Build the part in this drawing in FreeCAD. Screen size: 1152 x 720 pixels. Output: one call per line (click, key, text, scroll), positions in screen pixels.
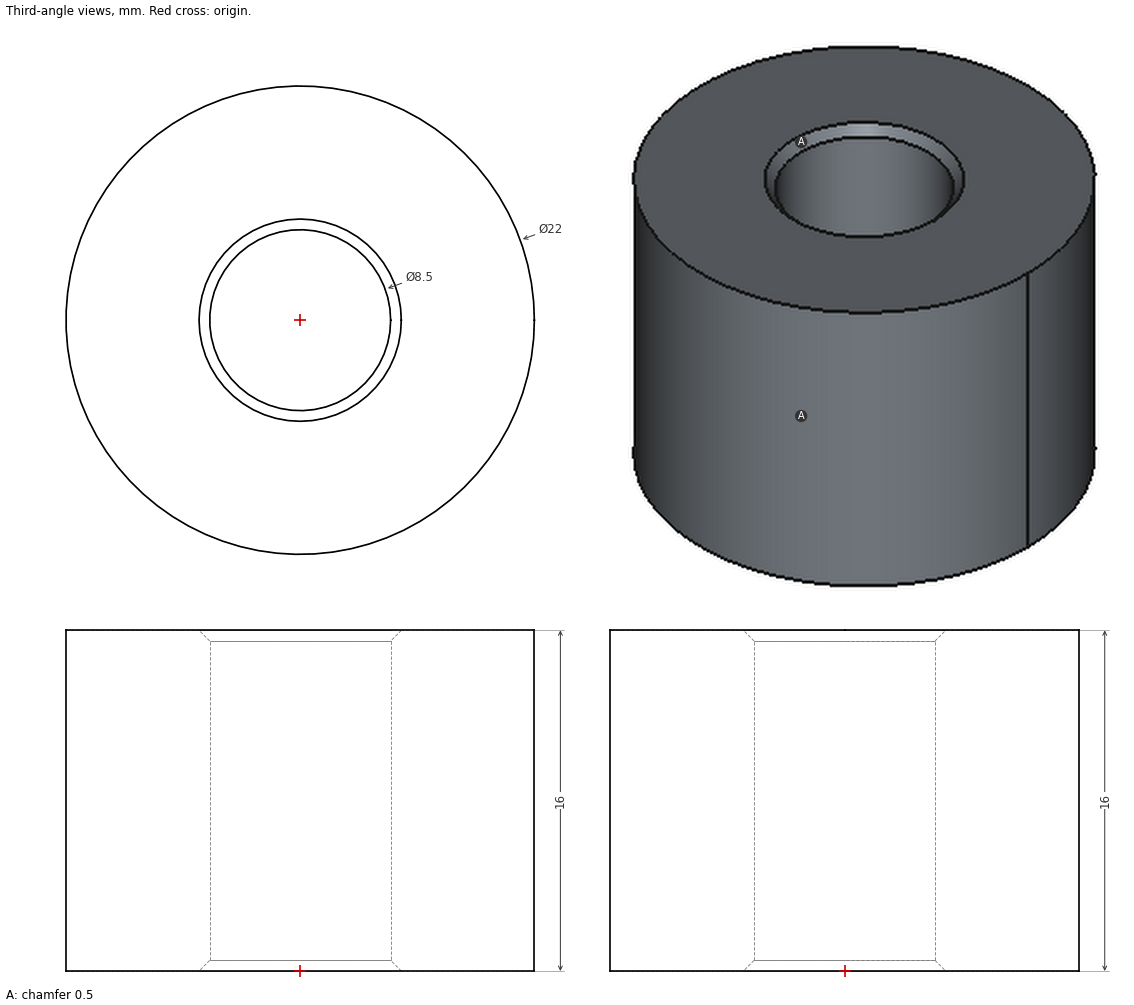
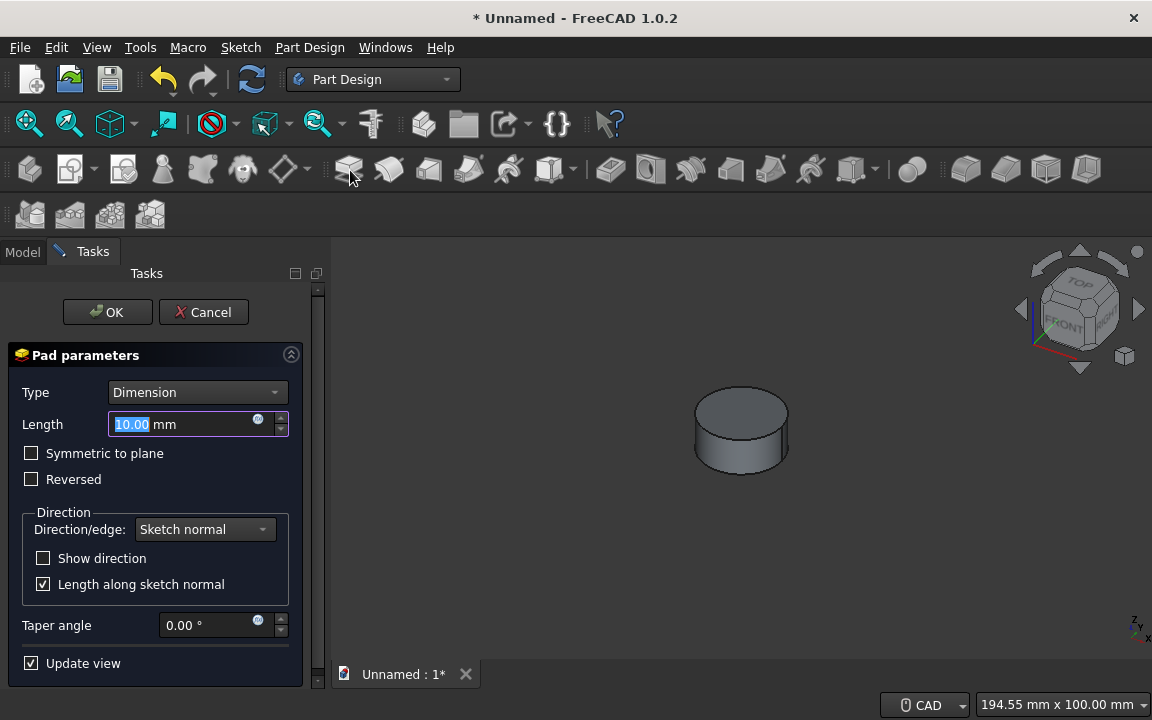
text(16)
key(Tab)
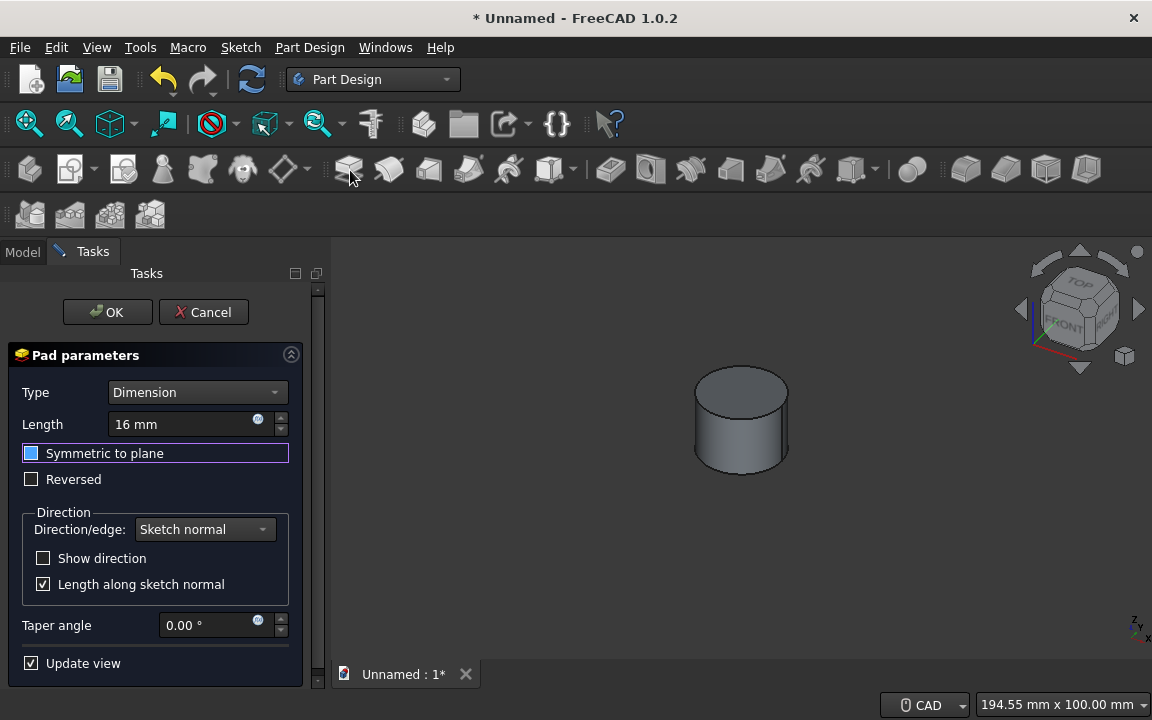
click(108, 312)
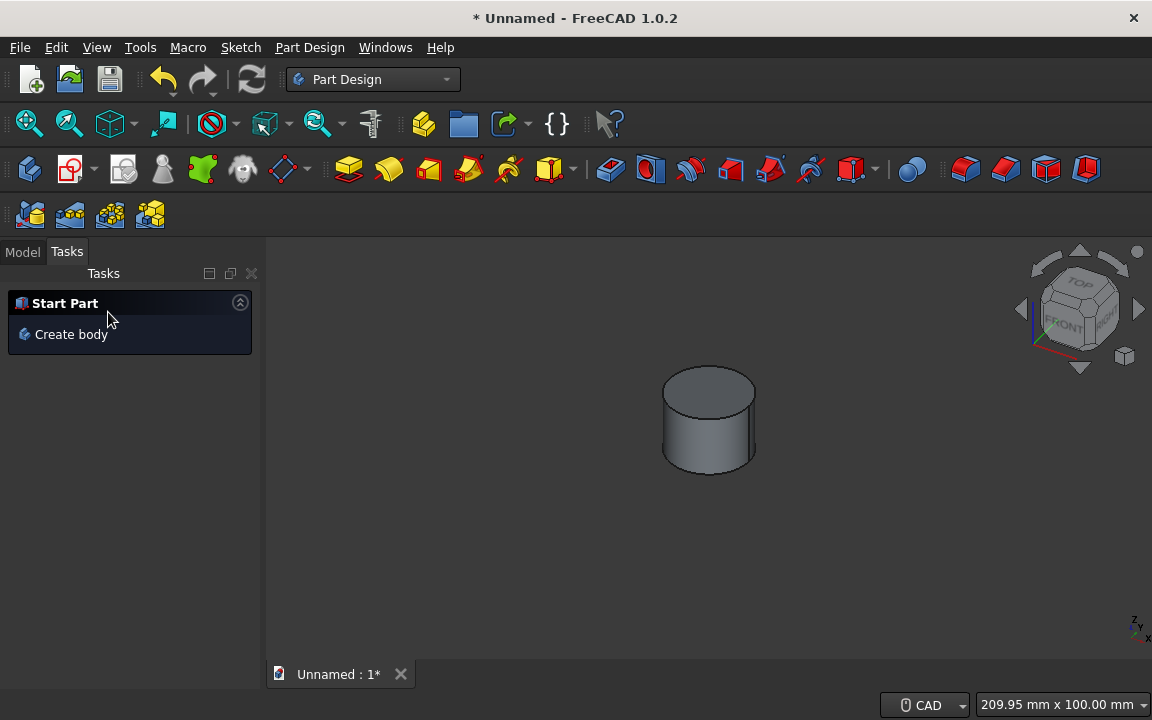
key(v)
key(f)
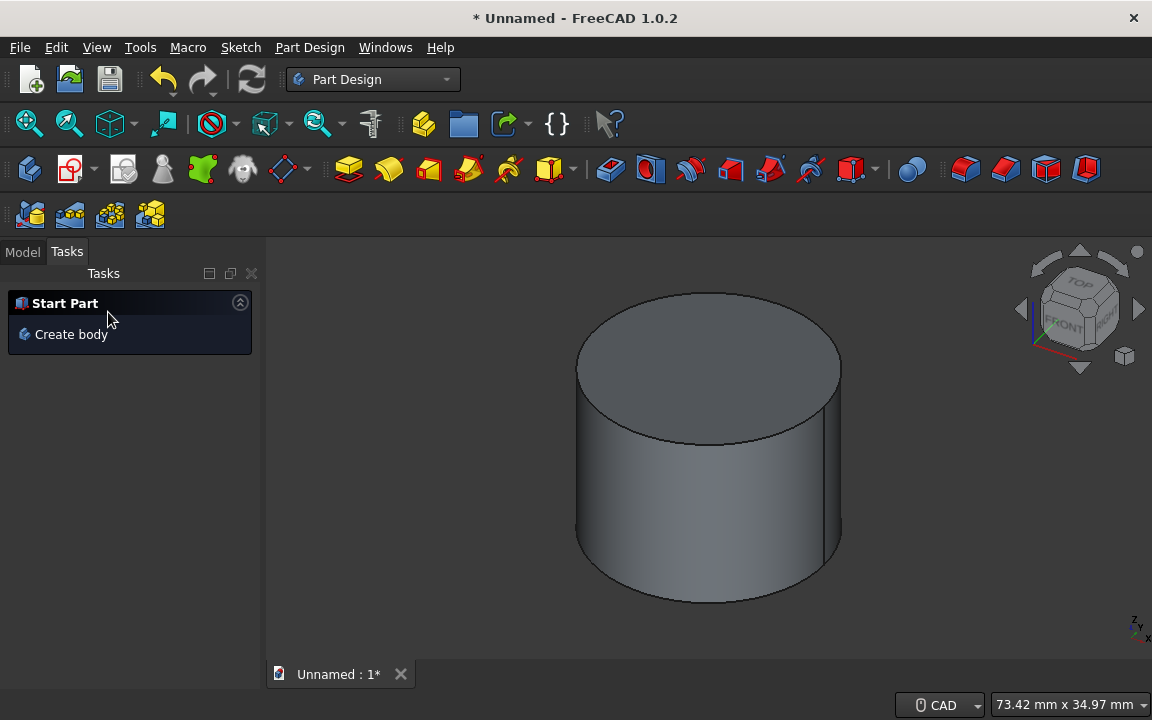
click(709, 368)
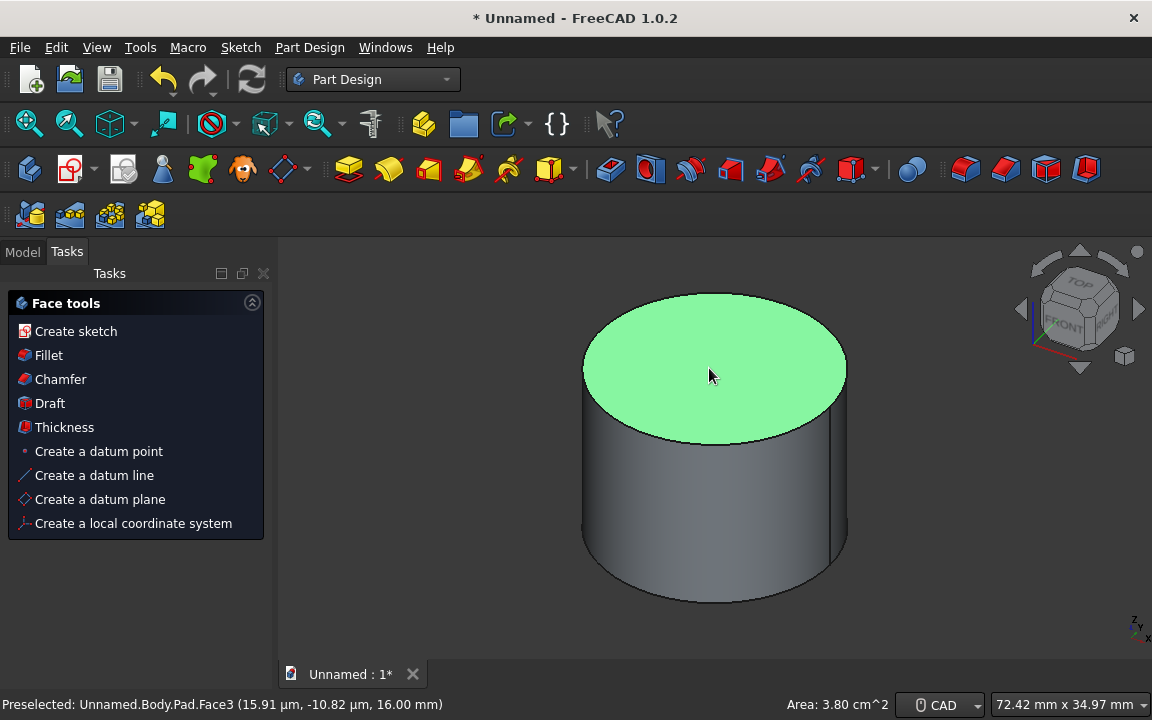
click(70, 170)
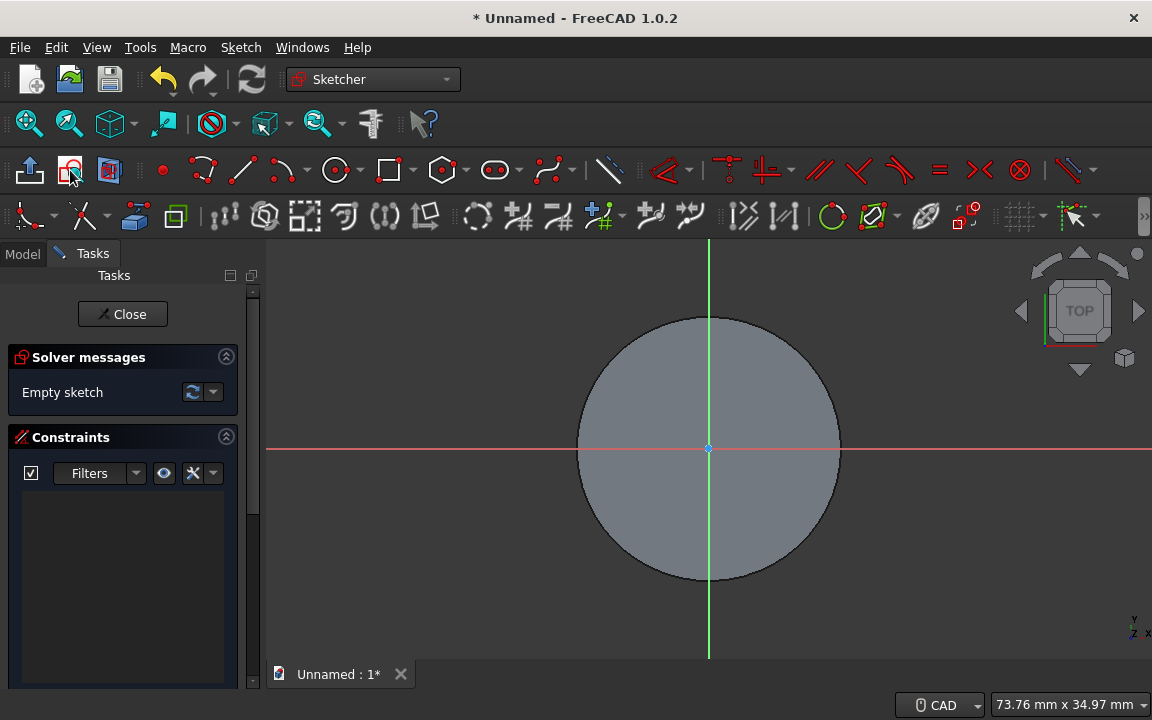
scroll(749, 449, up, 5)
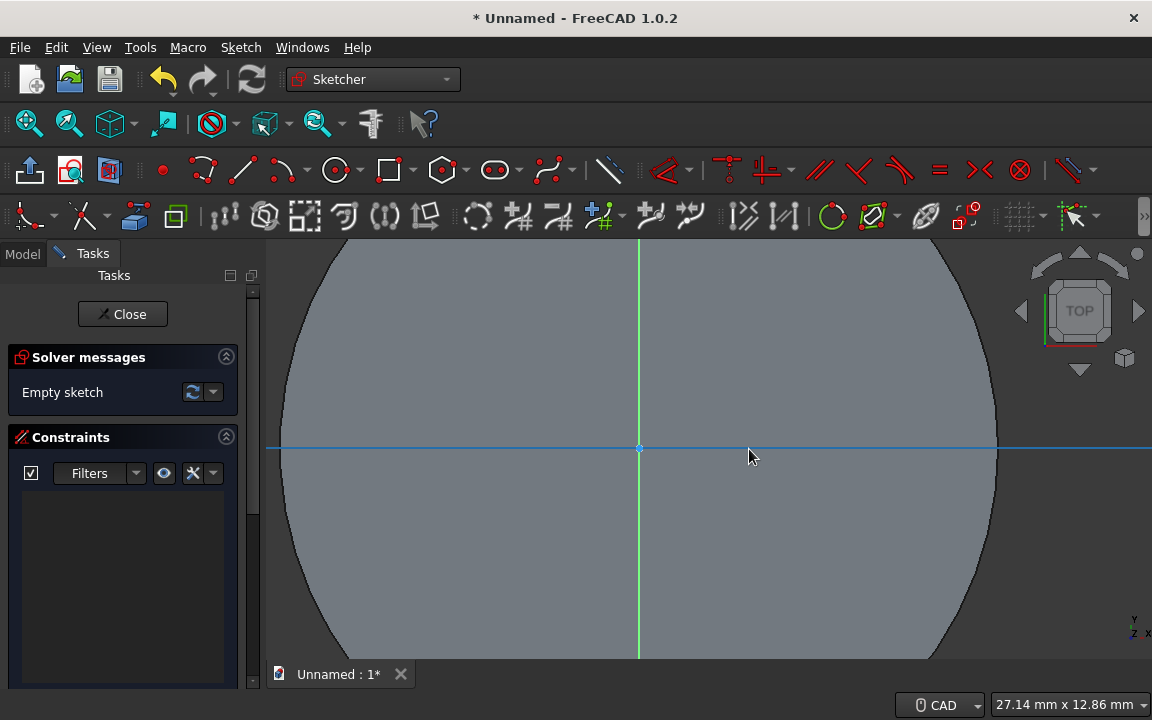
click(336, 170)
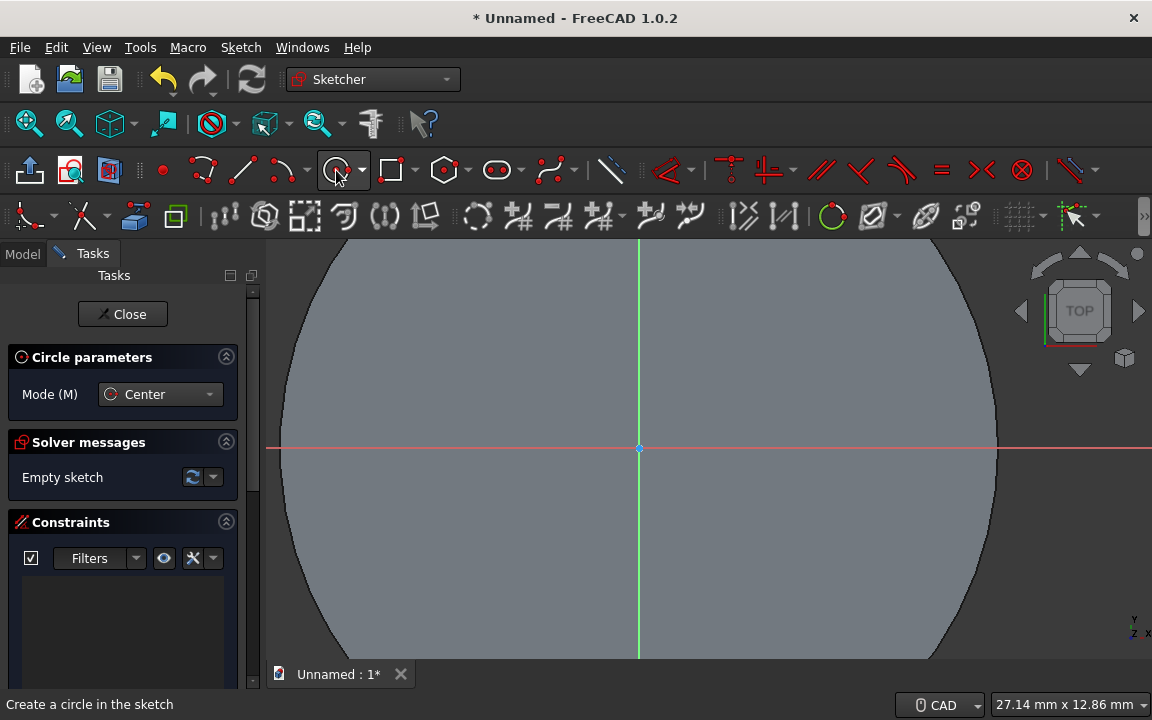
click(639, 448)
click(737, 350)
key(Escape)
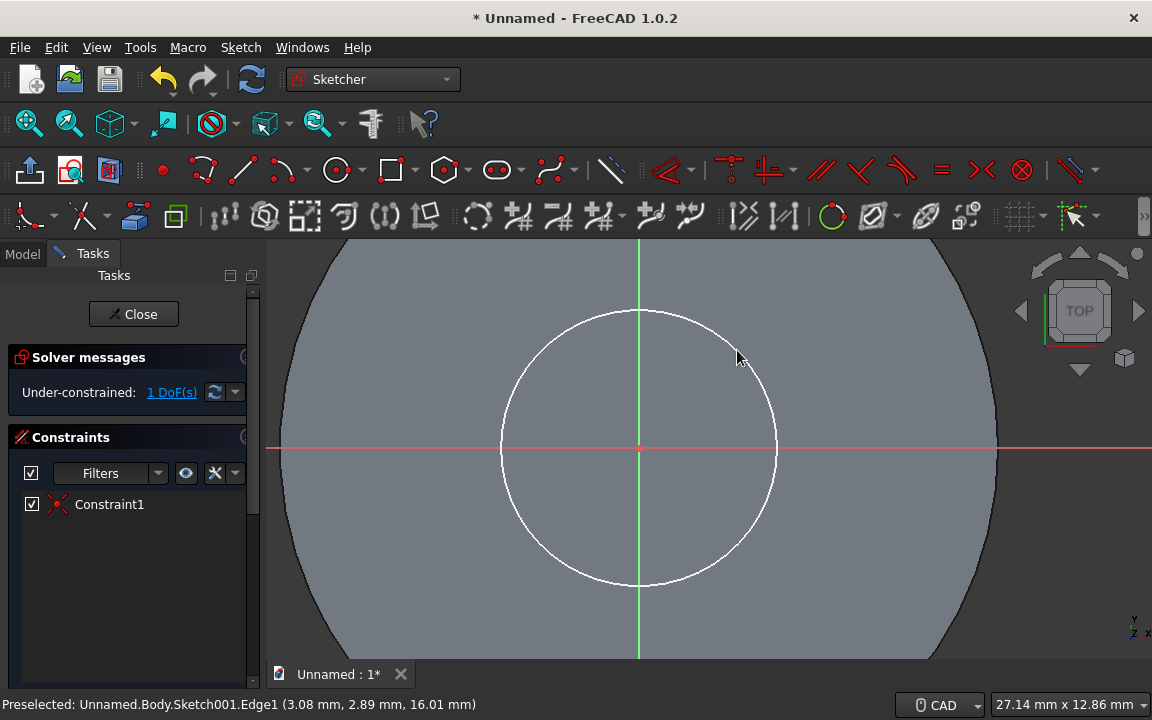
click(666, 170)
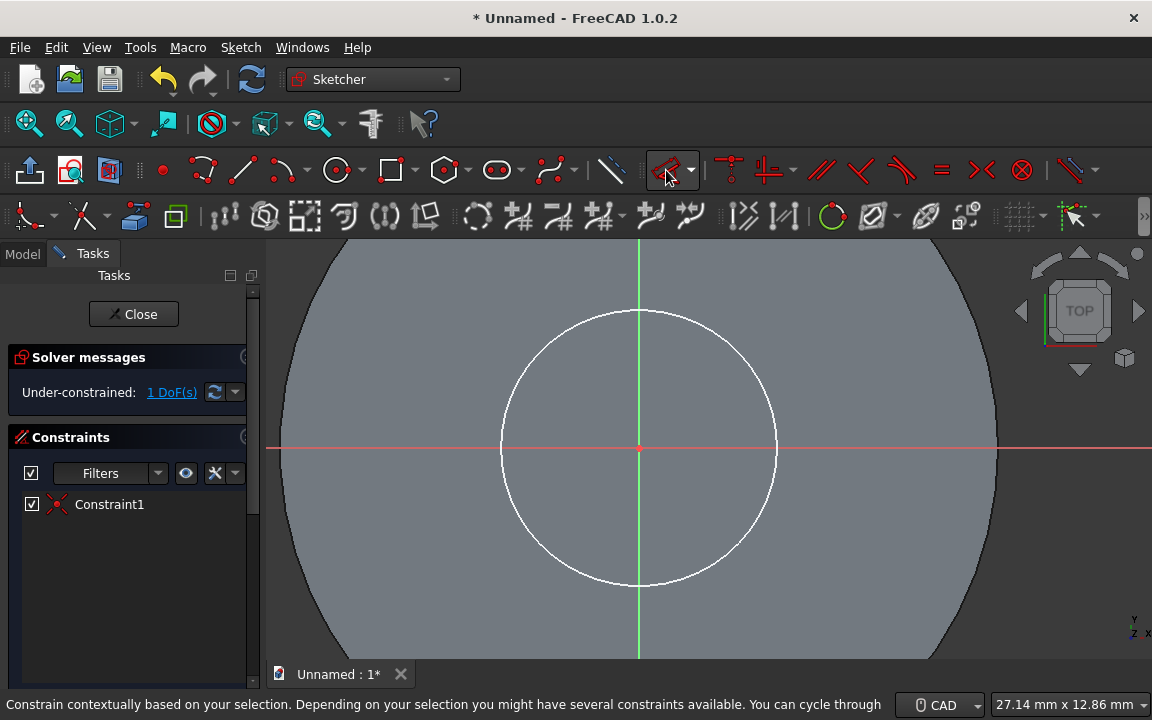
click(736, 350)
click(758, 327)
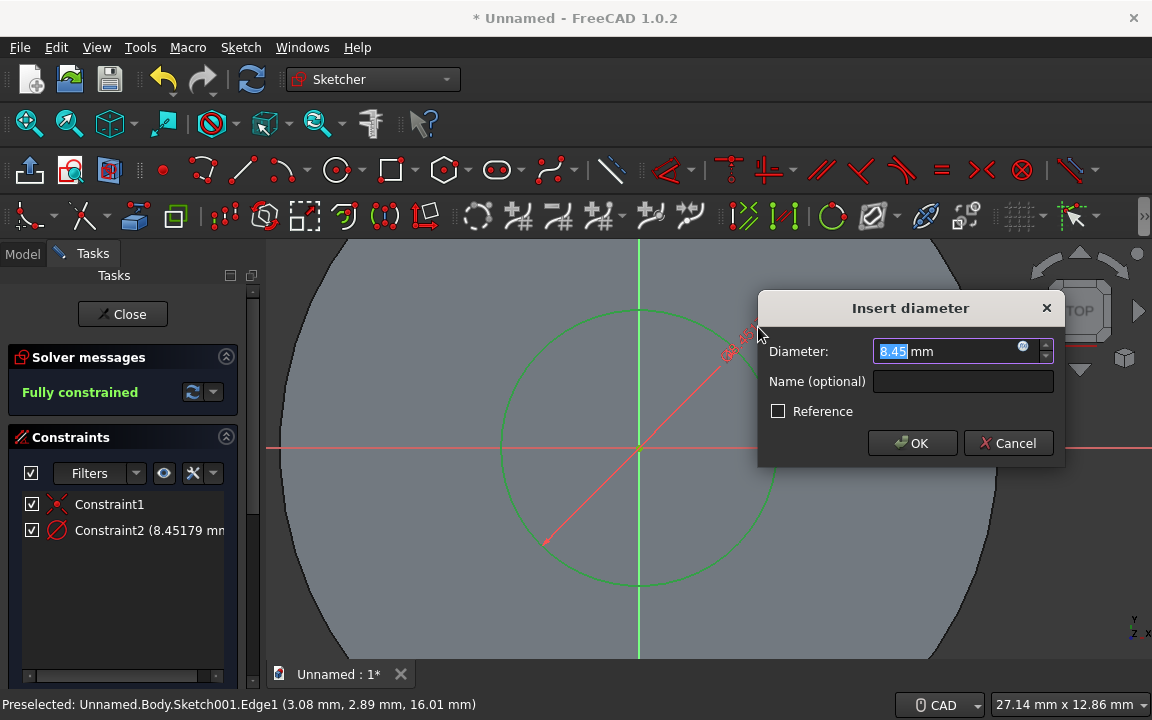
text(8.5)
key(Return)
key(Escape)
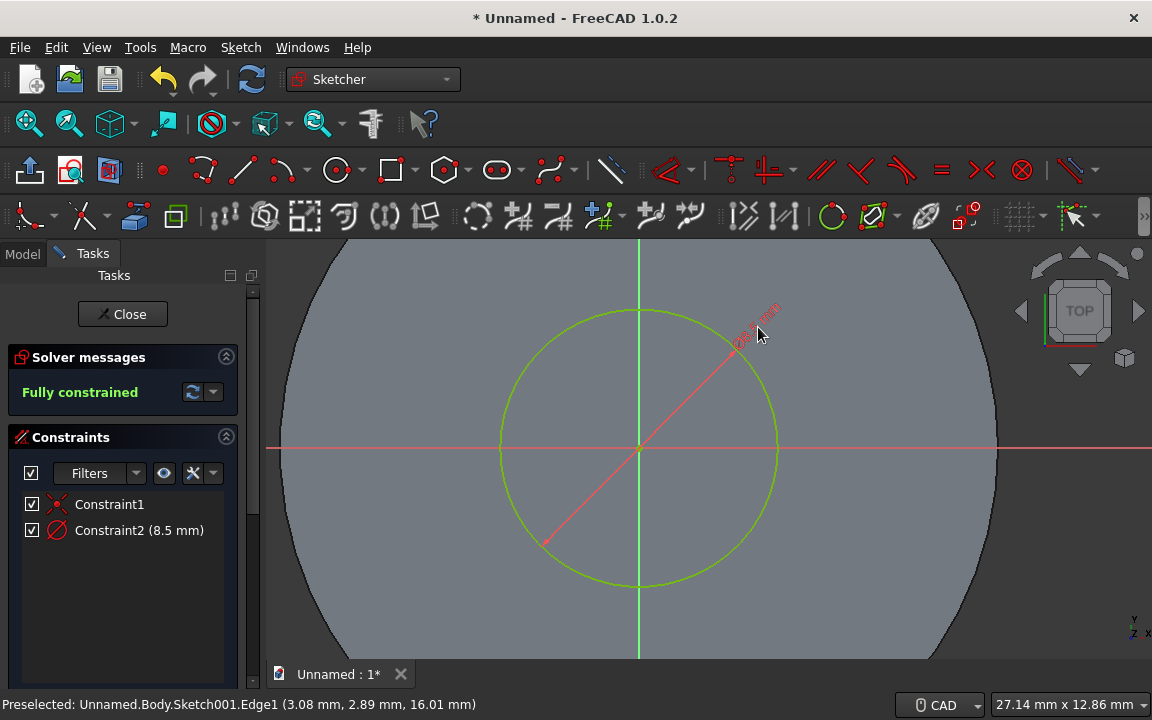
click(123, 314)